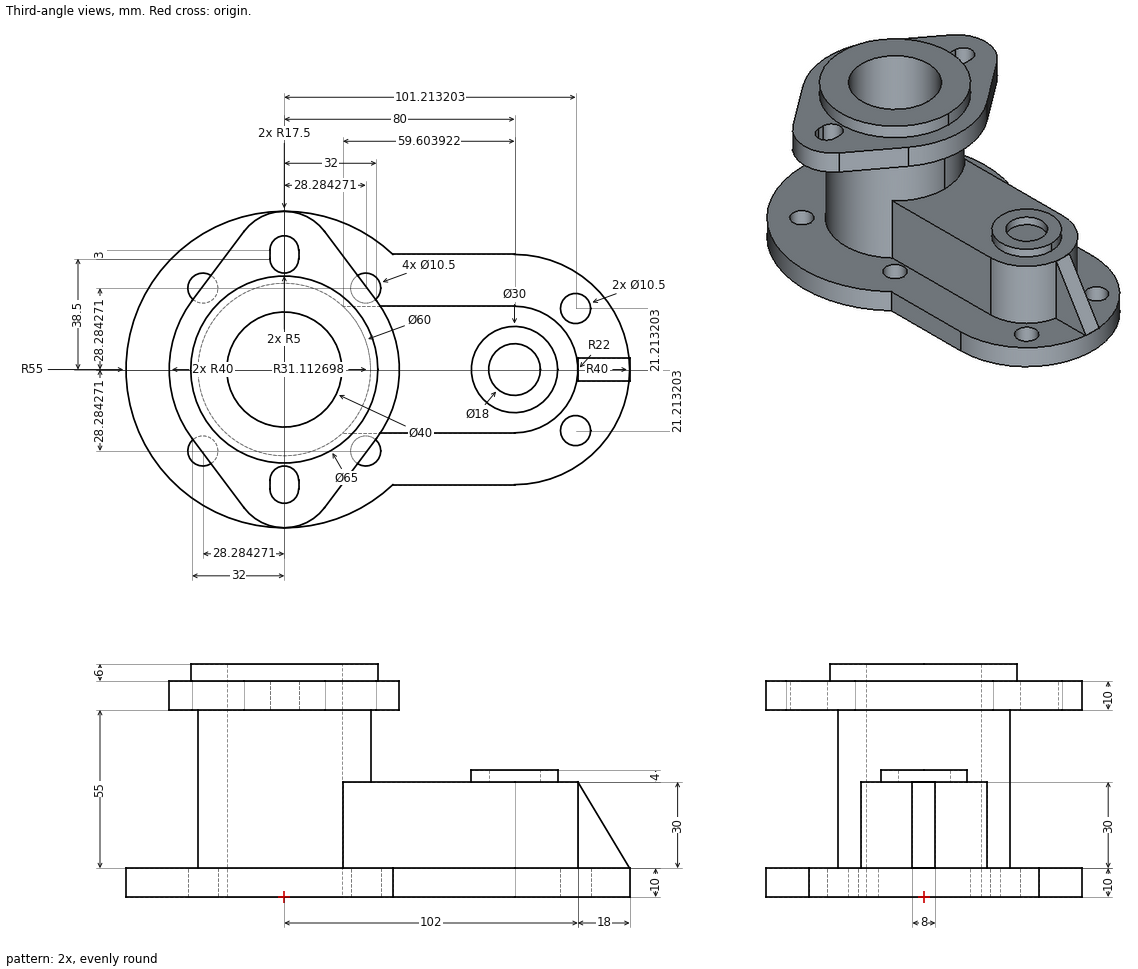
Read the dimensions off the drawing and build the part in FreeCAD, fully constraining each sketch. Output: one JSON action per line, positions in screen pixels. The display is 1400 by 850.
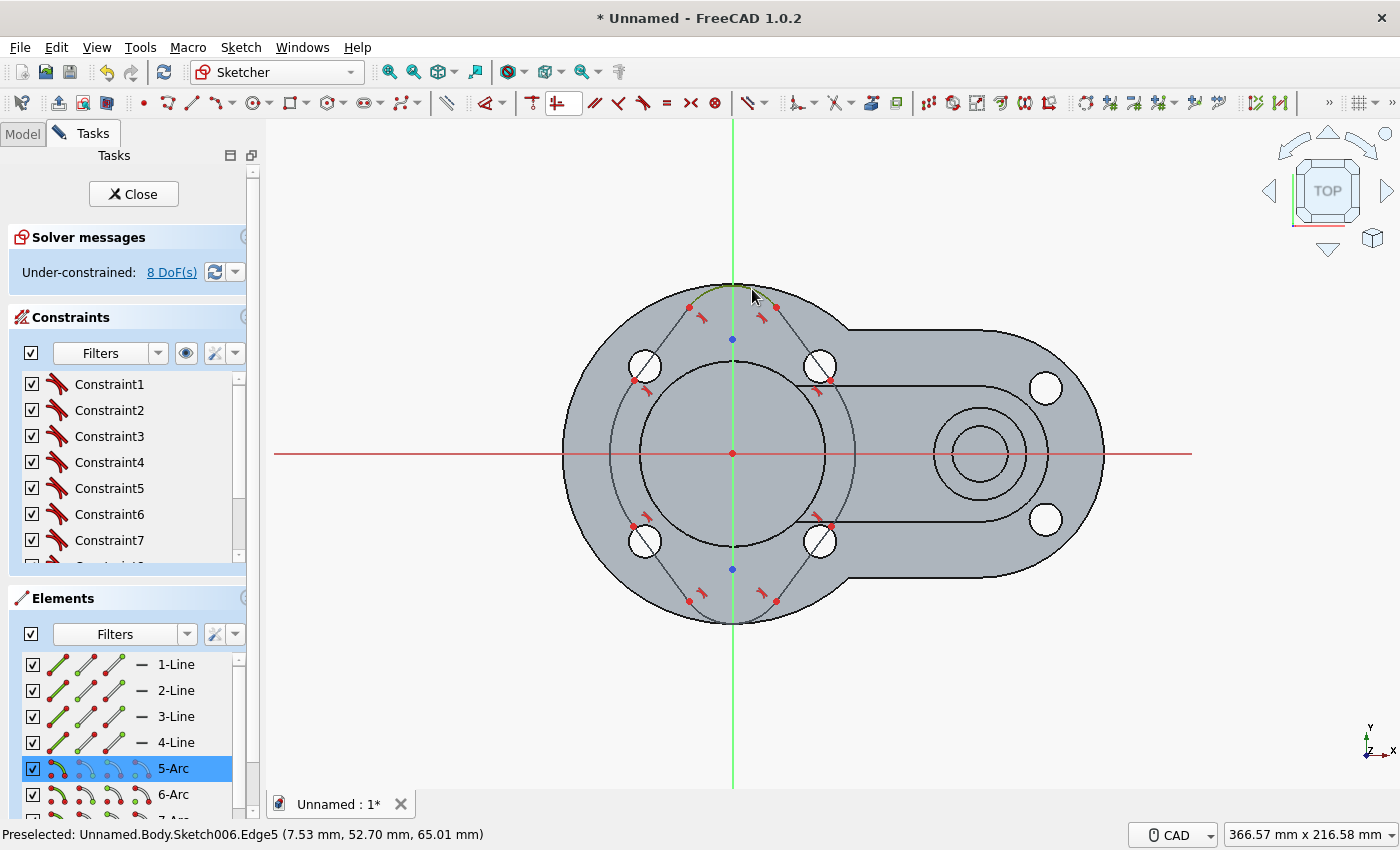
{"action": "left_click", "coordinate": [713, 620]}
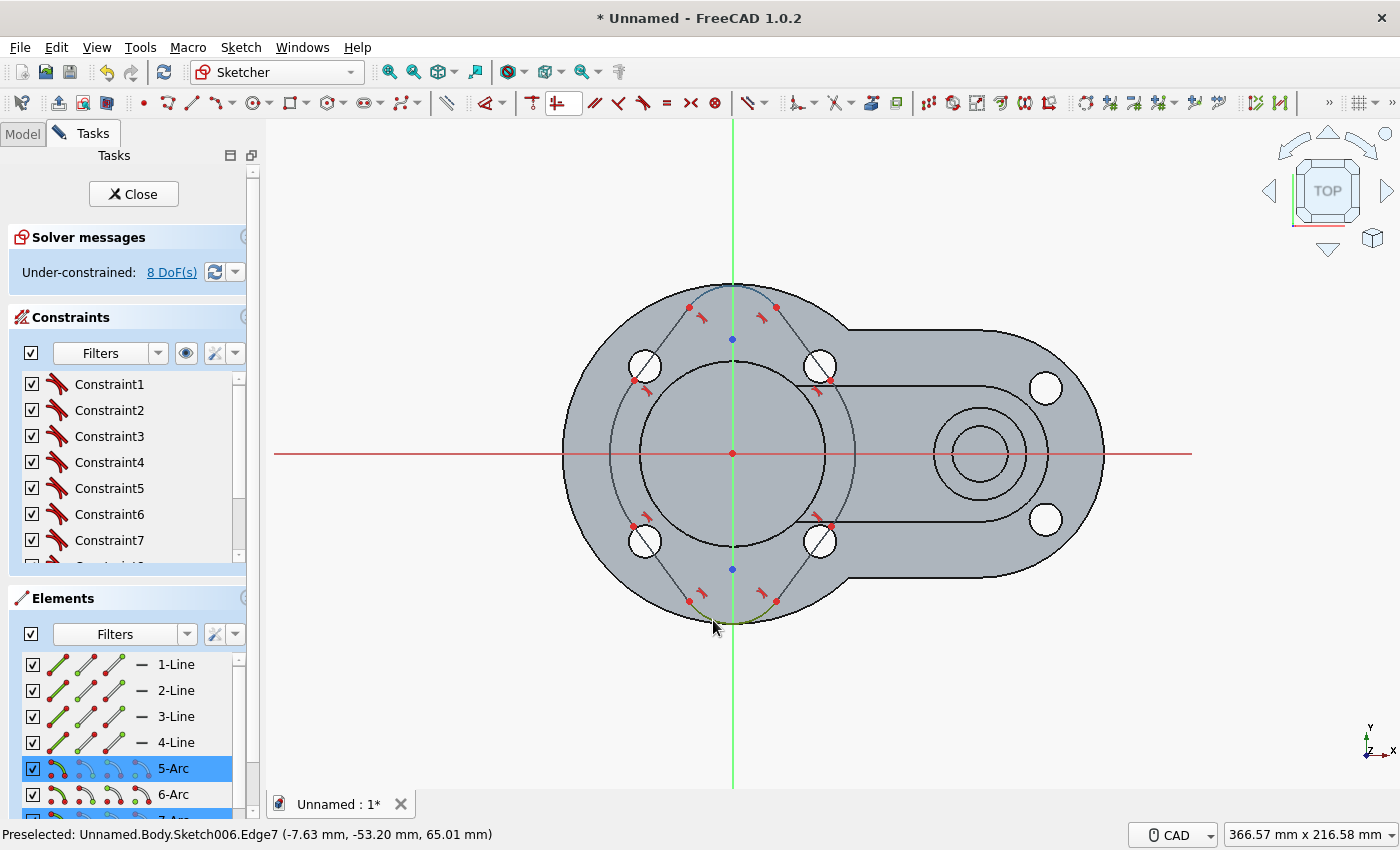
{"action": "left_click", "coordinate": [668, 104]}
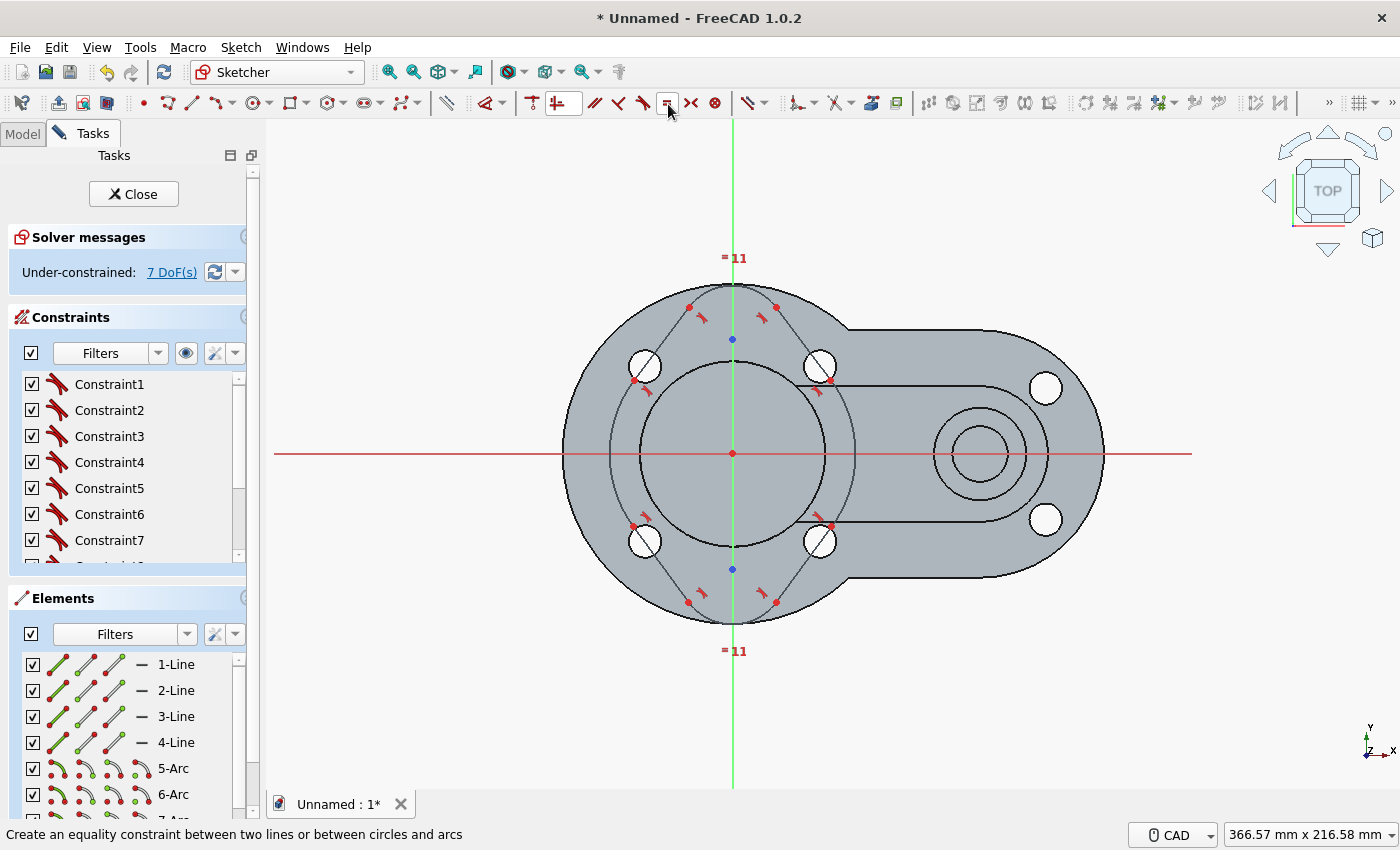
{"action": "left_click", "coordinate": [614, 422]}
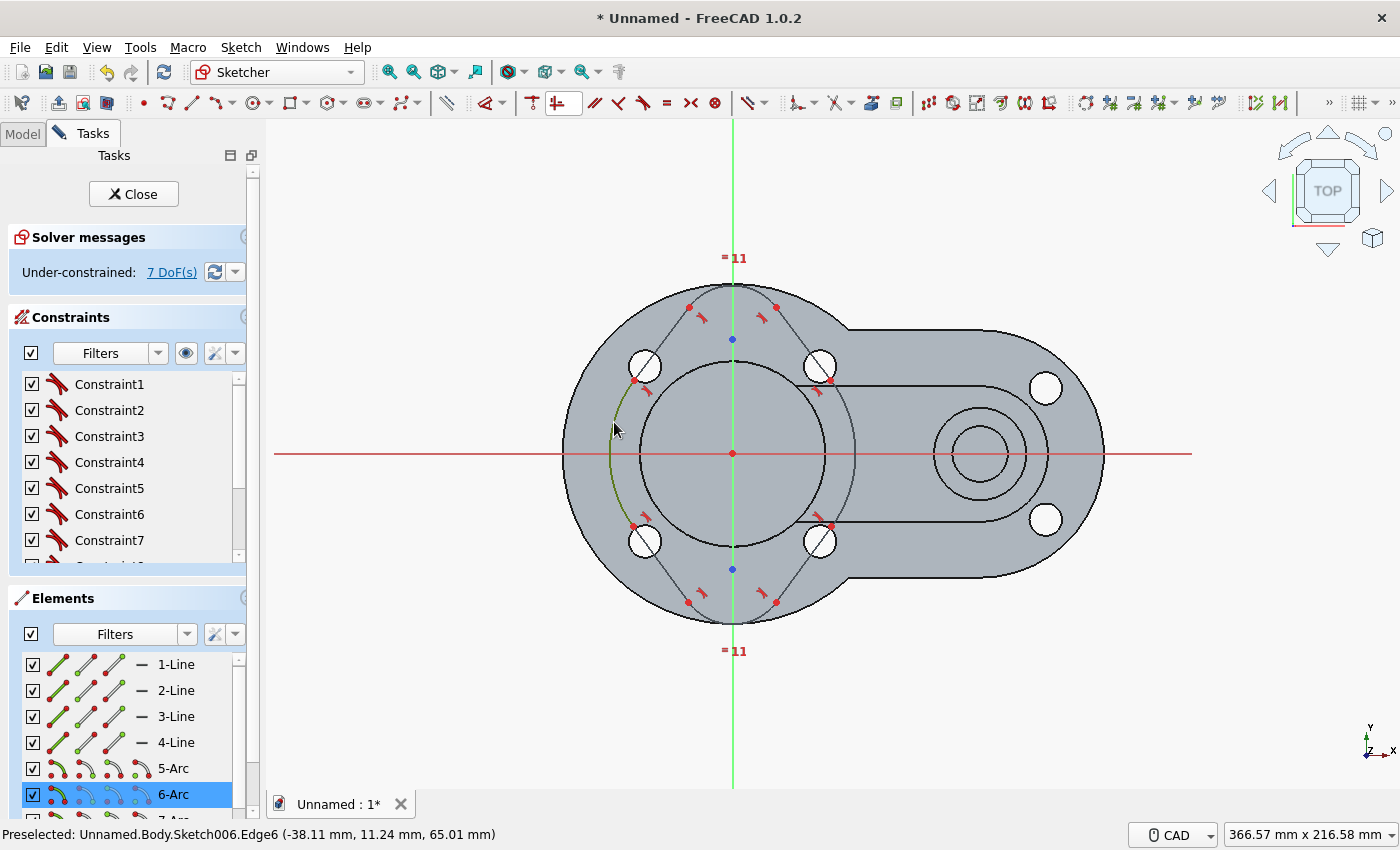
{"action": "left_click", "coordinate": [852, 484]}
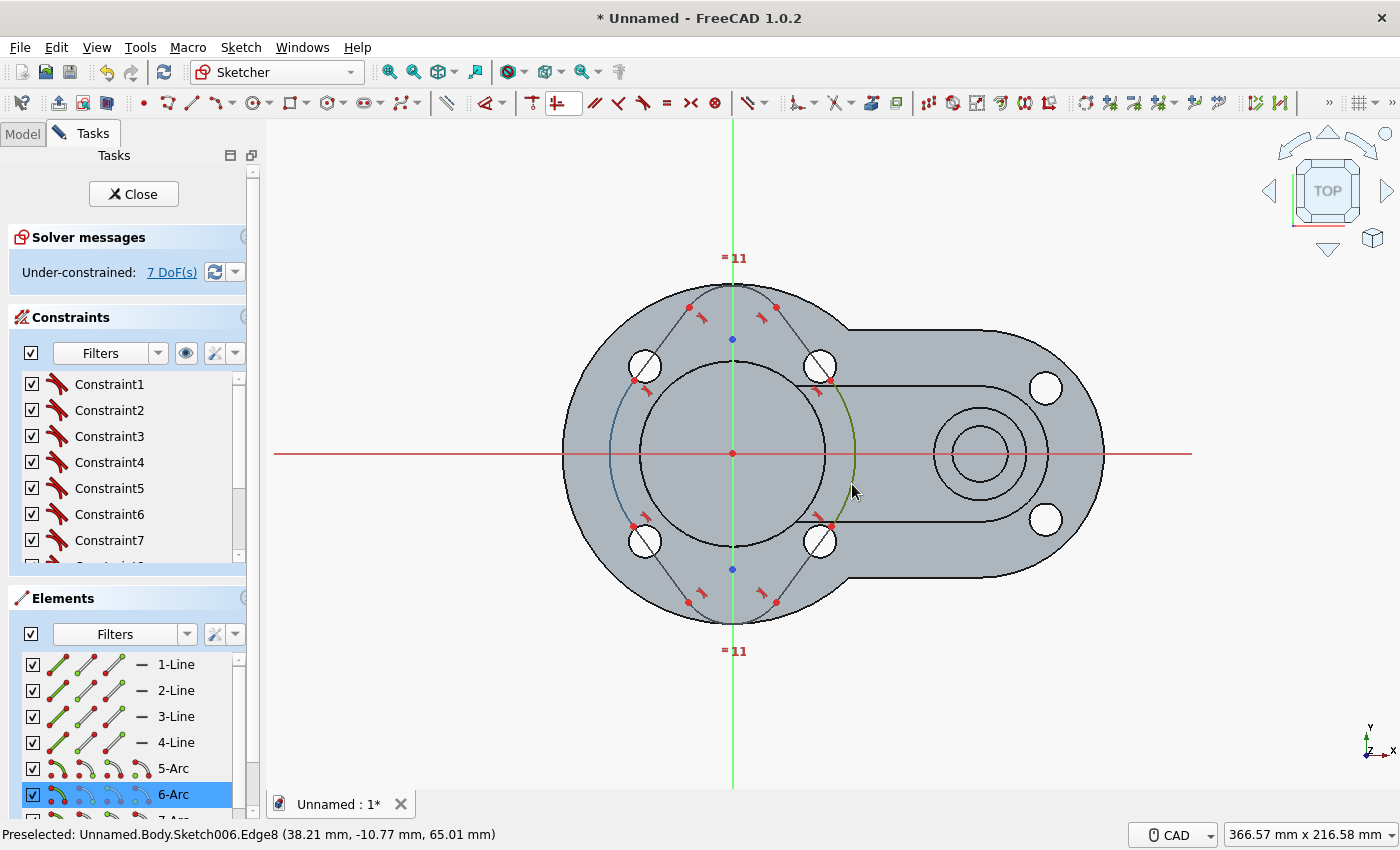
{"action": "key", "text": "e"}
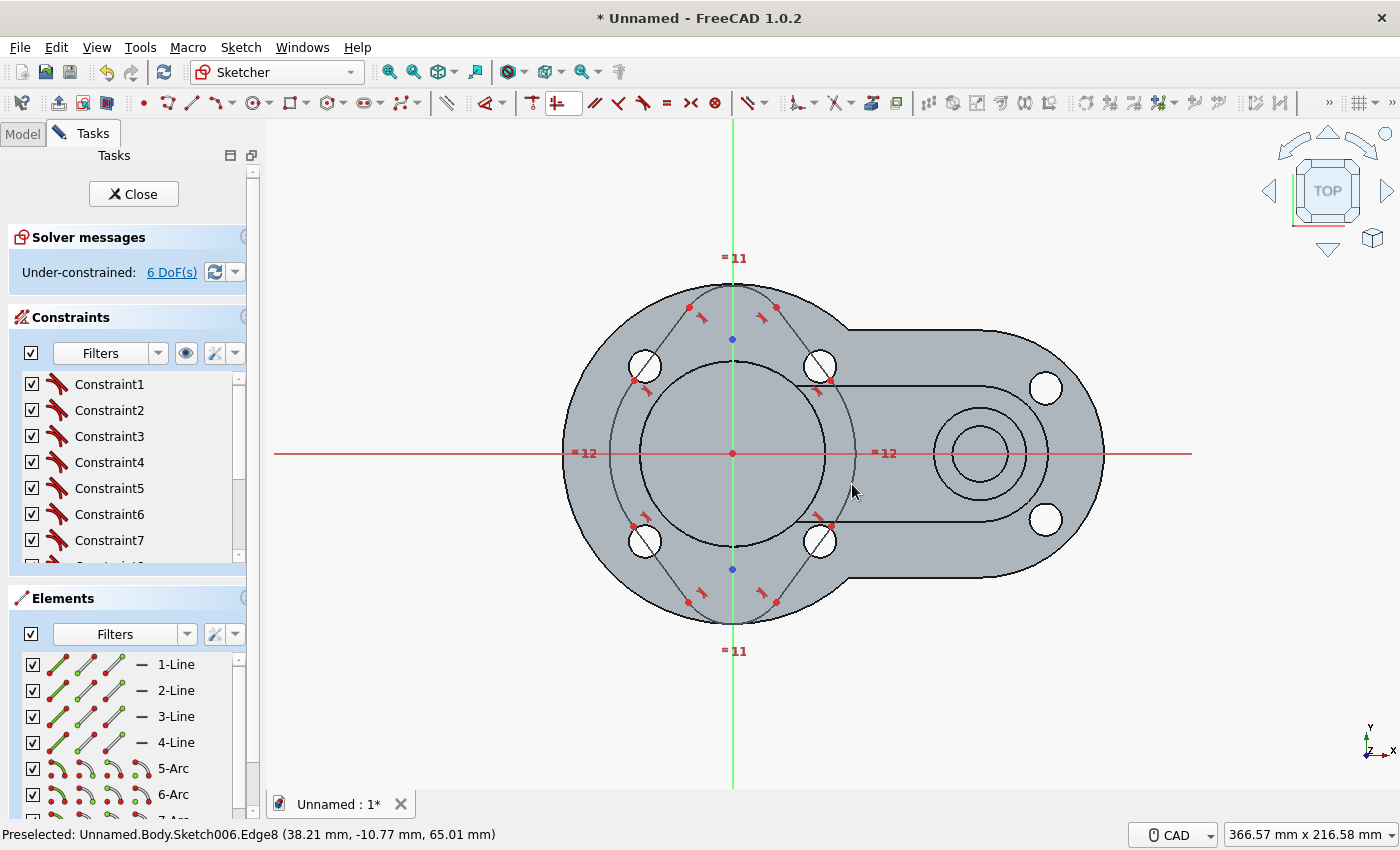
{"action": "left_click", "coordinate": [733, 340]}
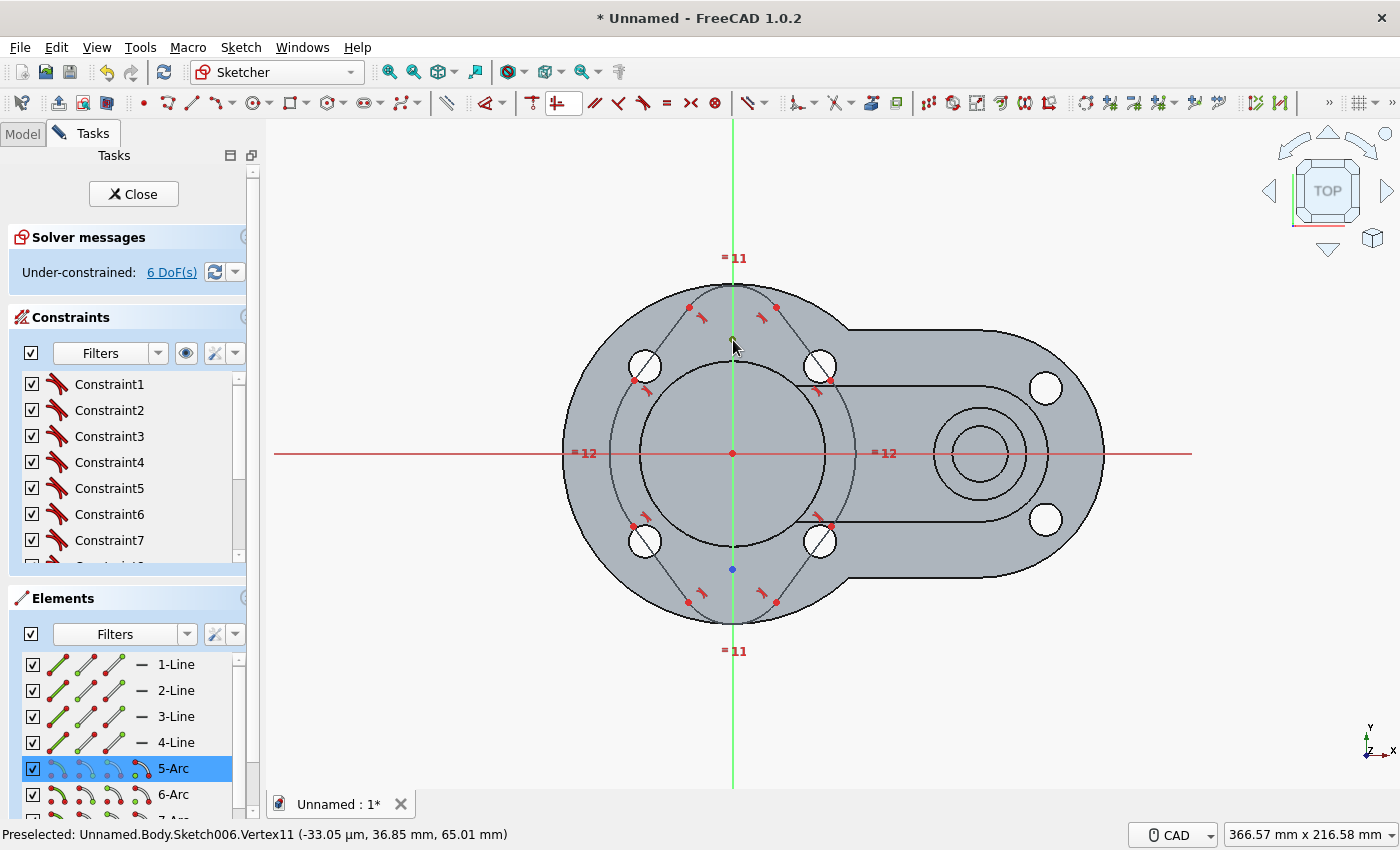
{"action": "left_click", "coordinate": [733, 717]}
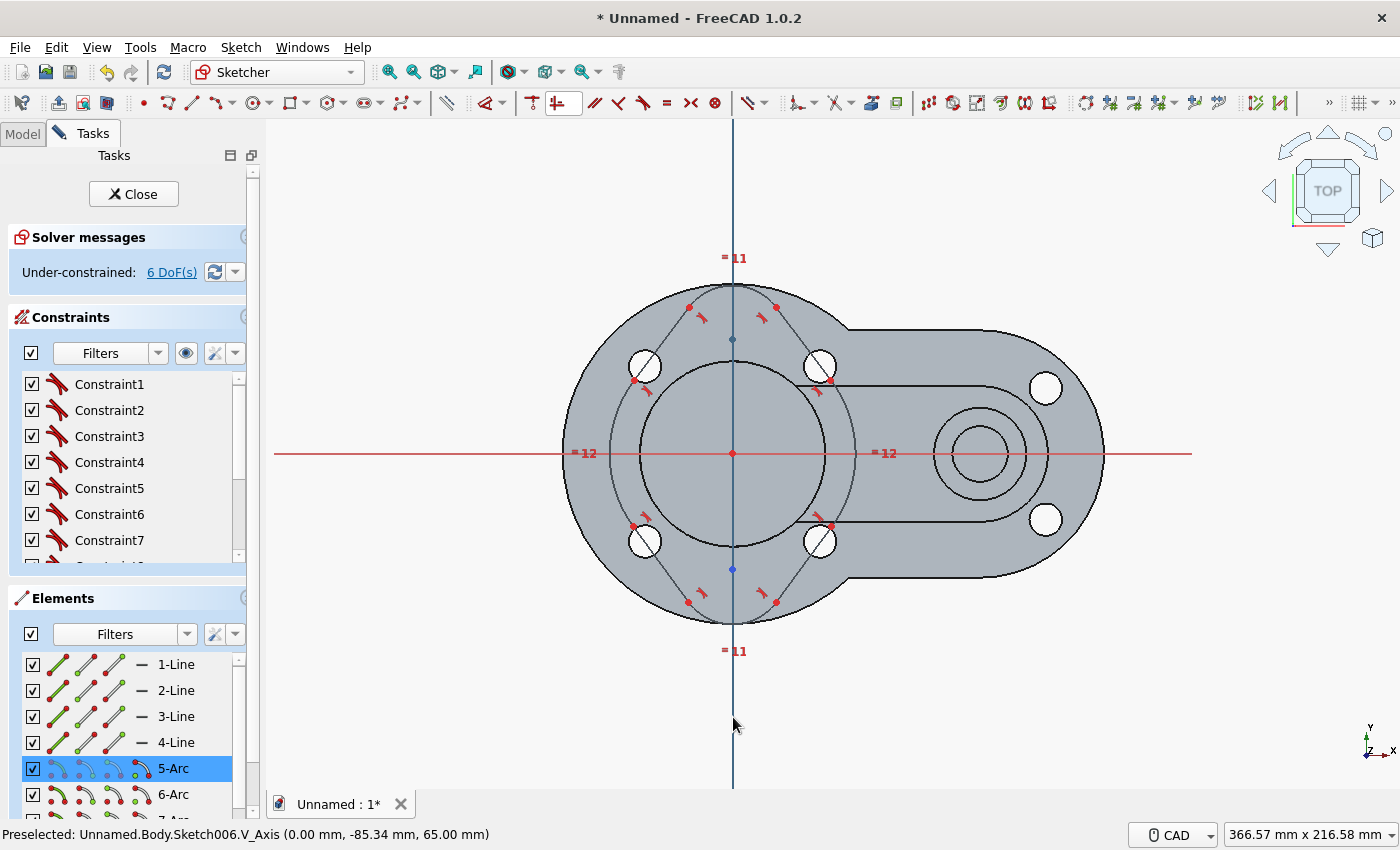
{"action": "key", "text": "c"}